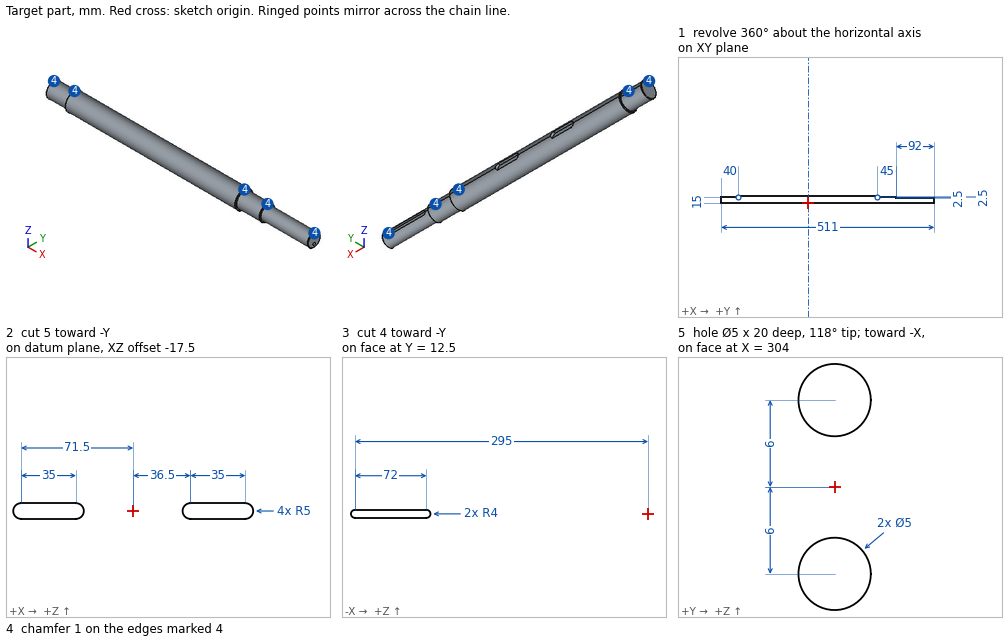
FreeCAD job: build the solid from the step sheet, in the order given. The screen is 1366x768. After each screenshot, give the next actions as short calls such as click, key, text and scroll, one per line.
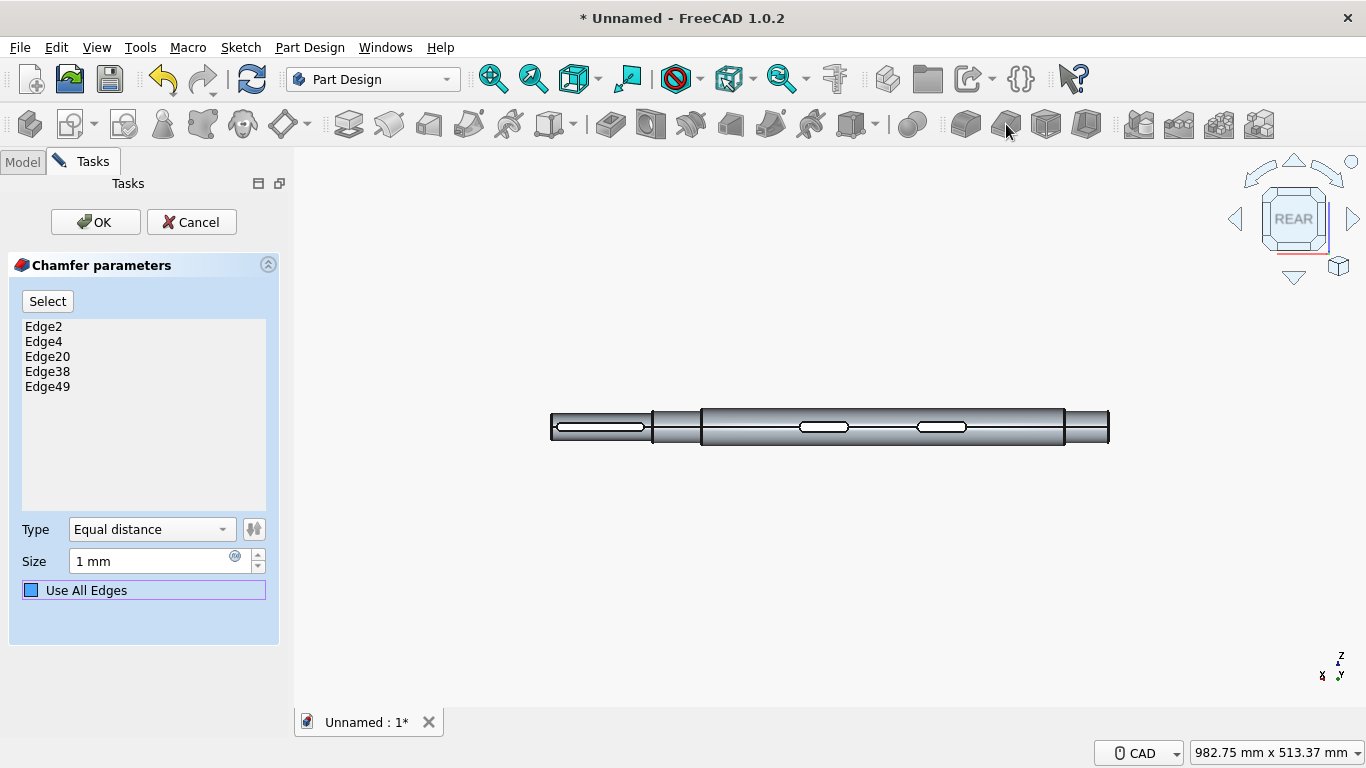
click(96, 222)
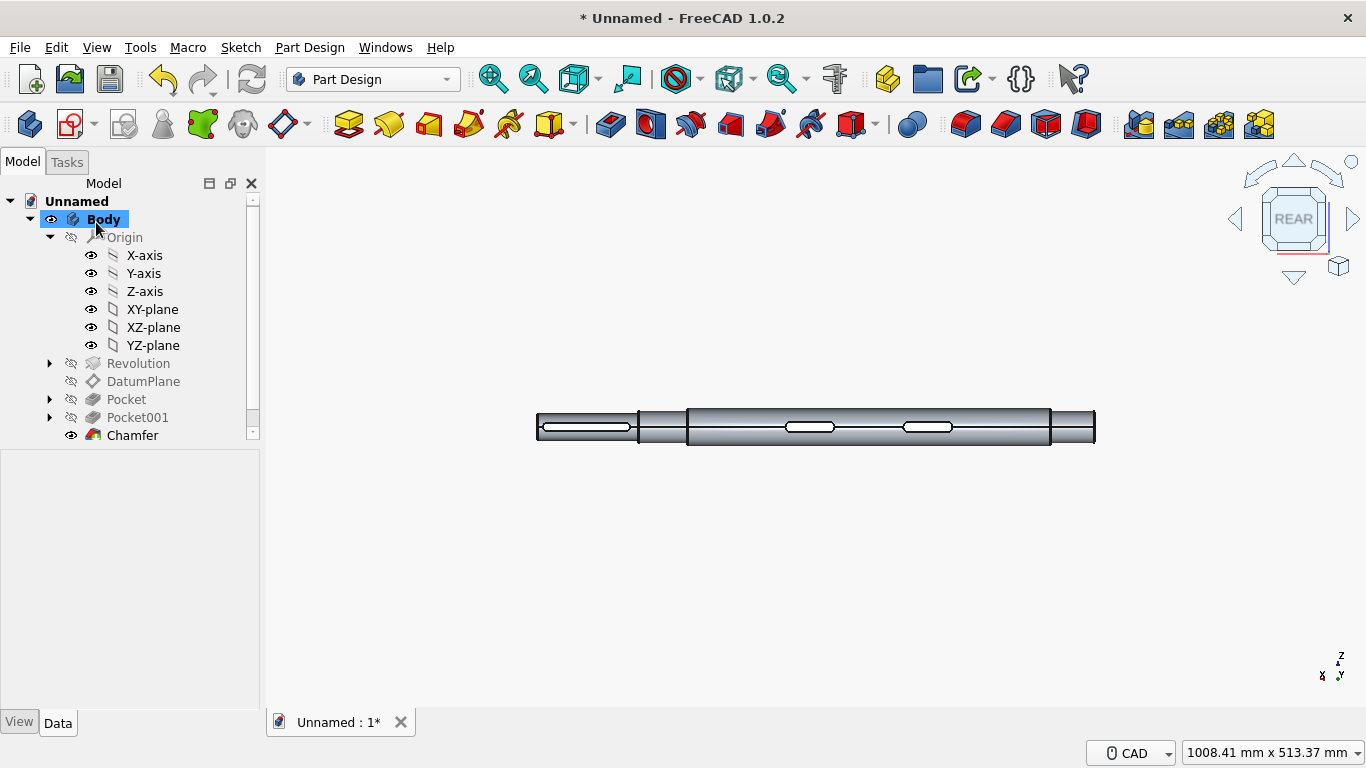
key(0)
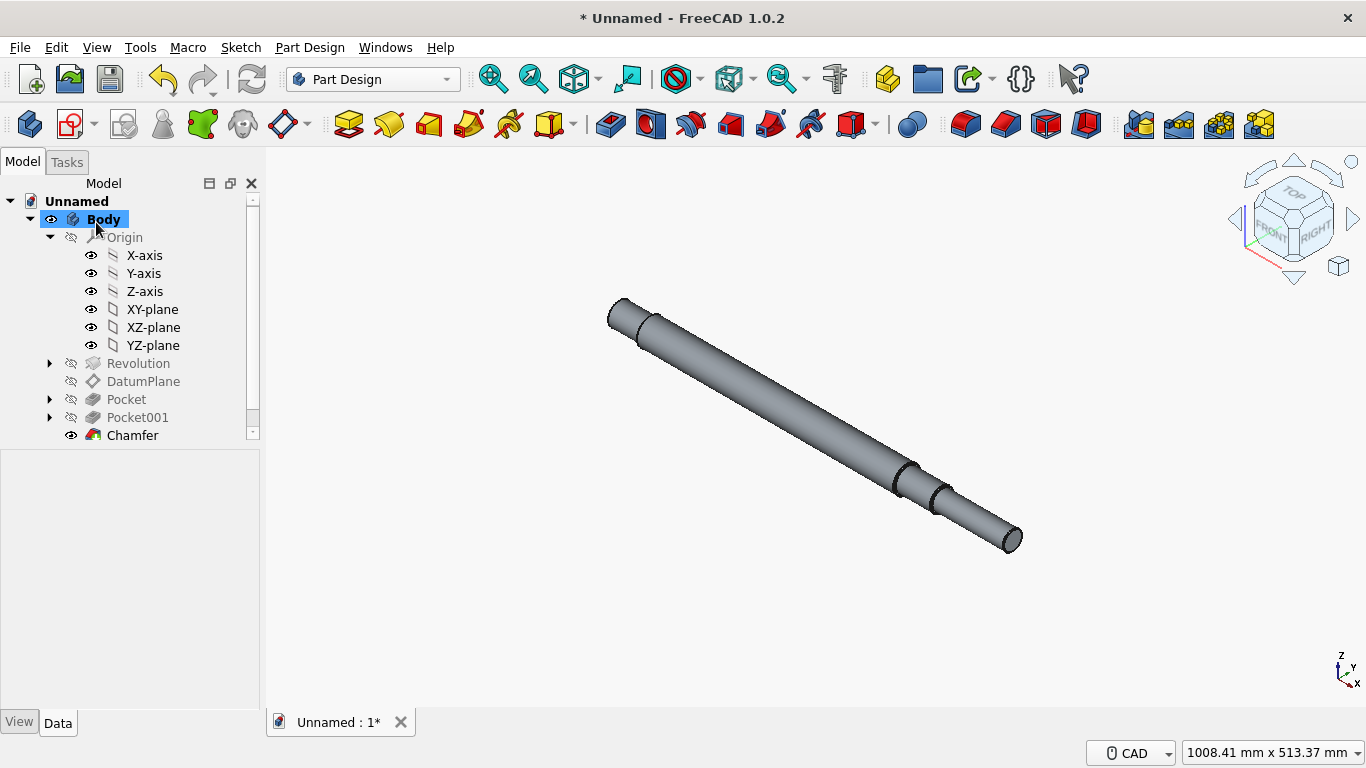
key(3)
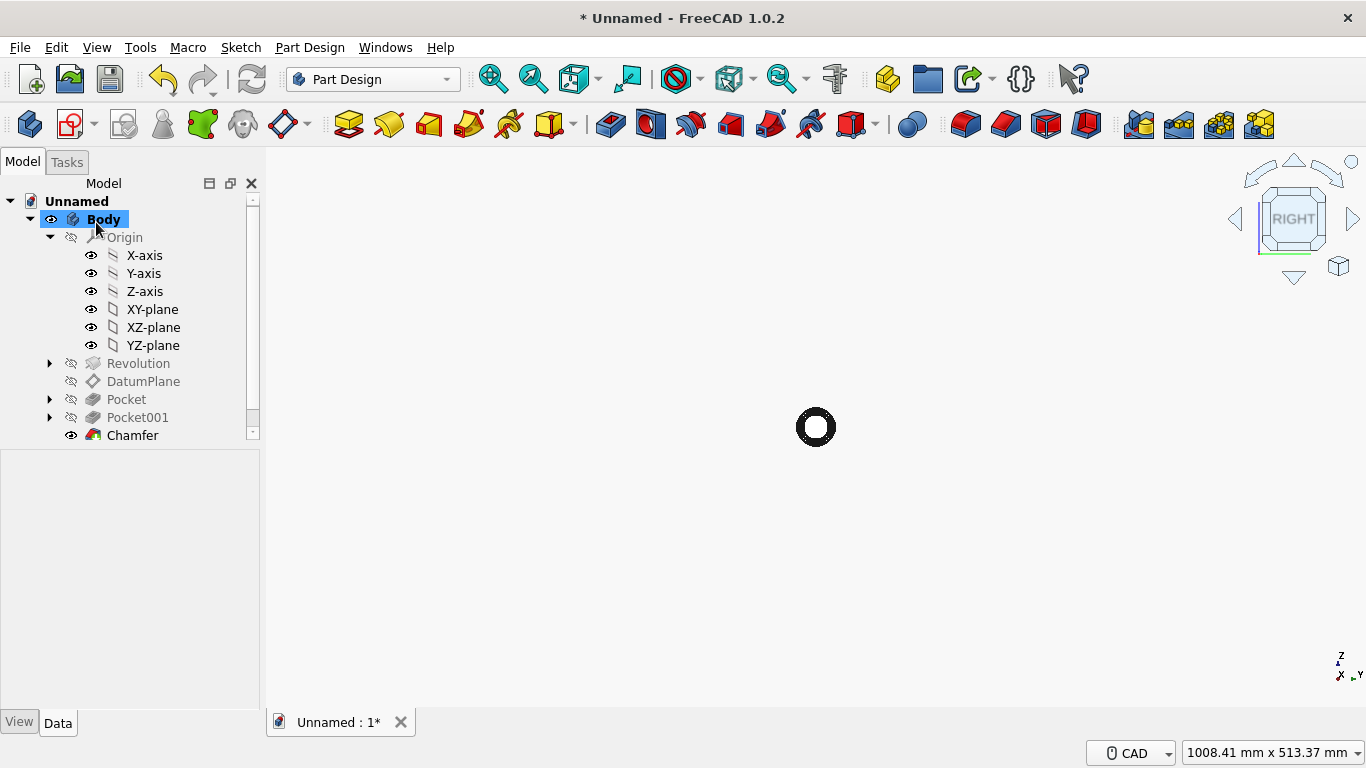
key(v)
key(f)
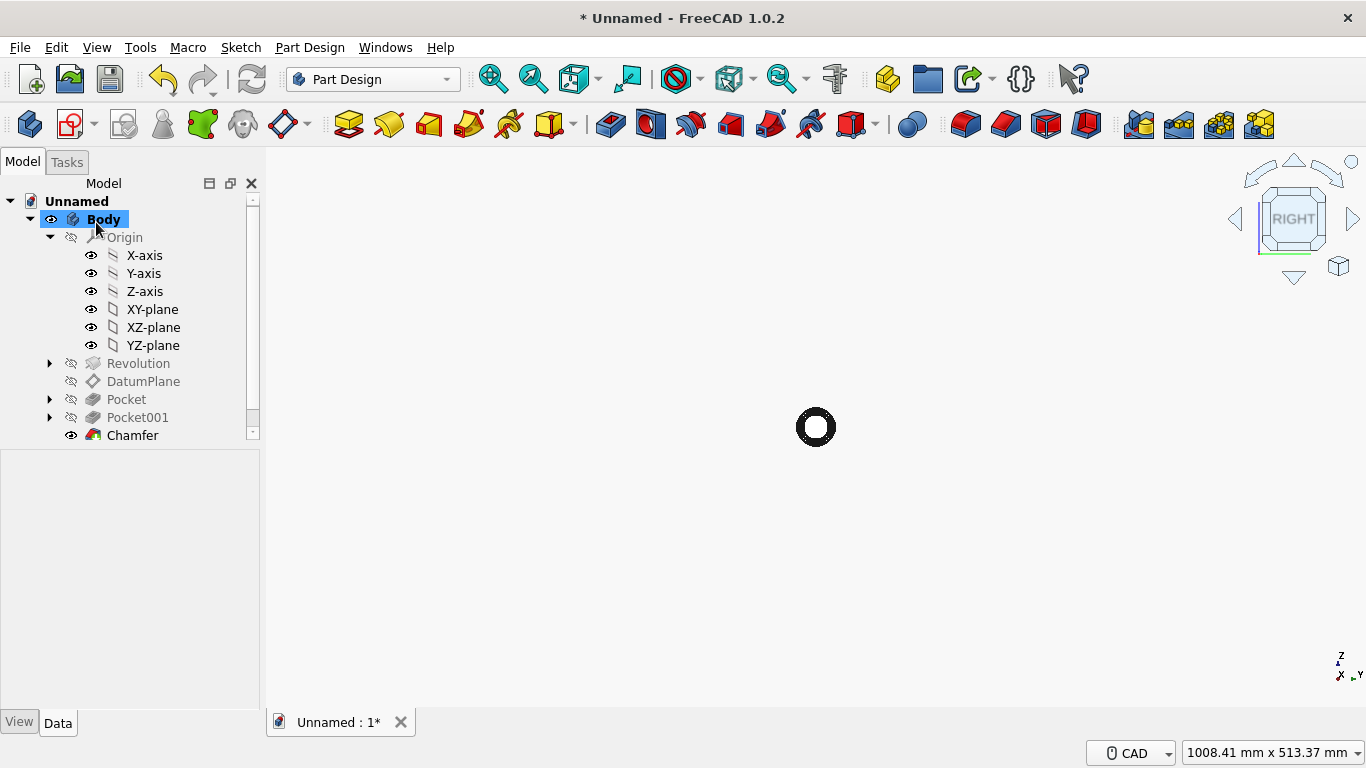
click(816, 426)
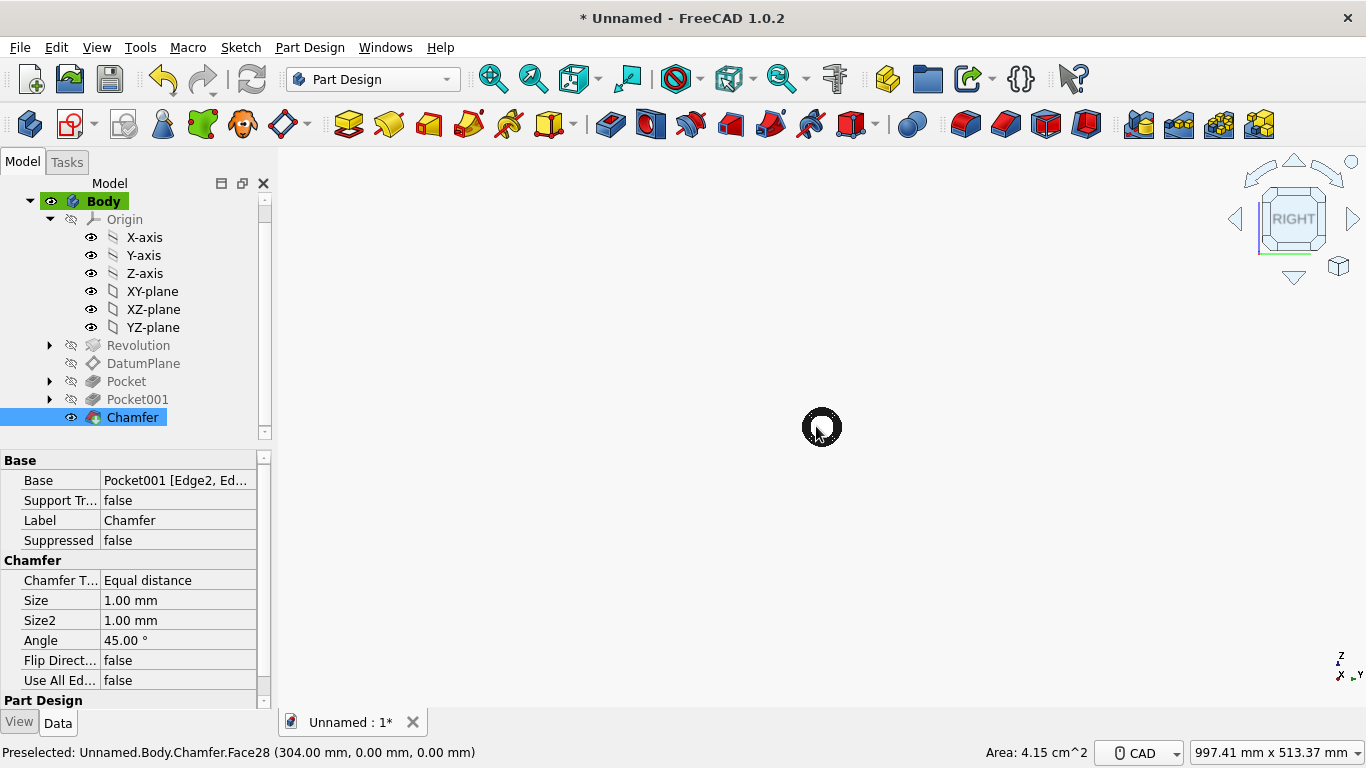
click(70, 124)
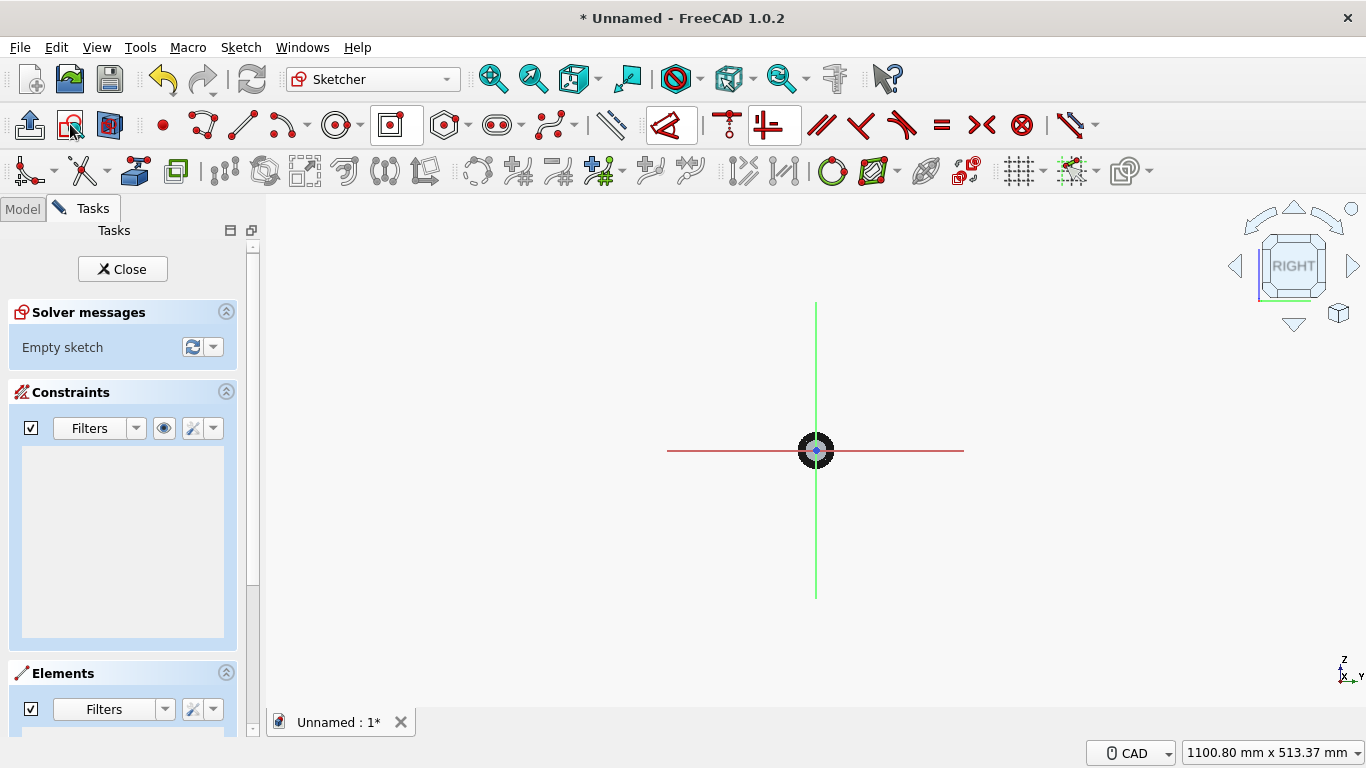
scroll(820, 451, up, 15)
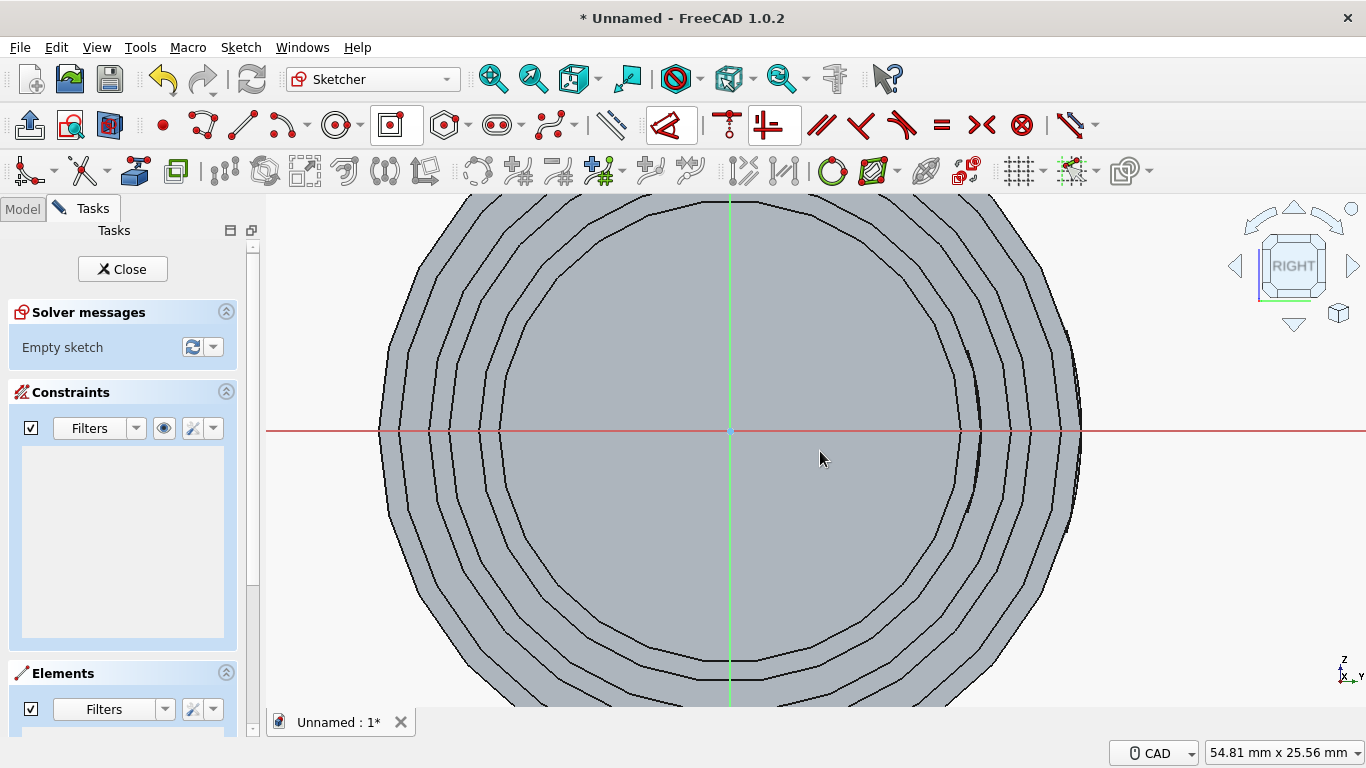
key(g)
key(c)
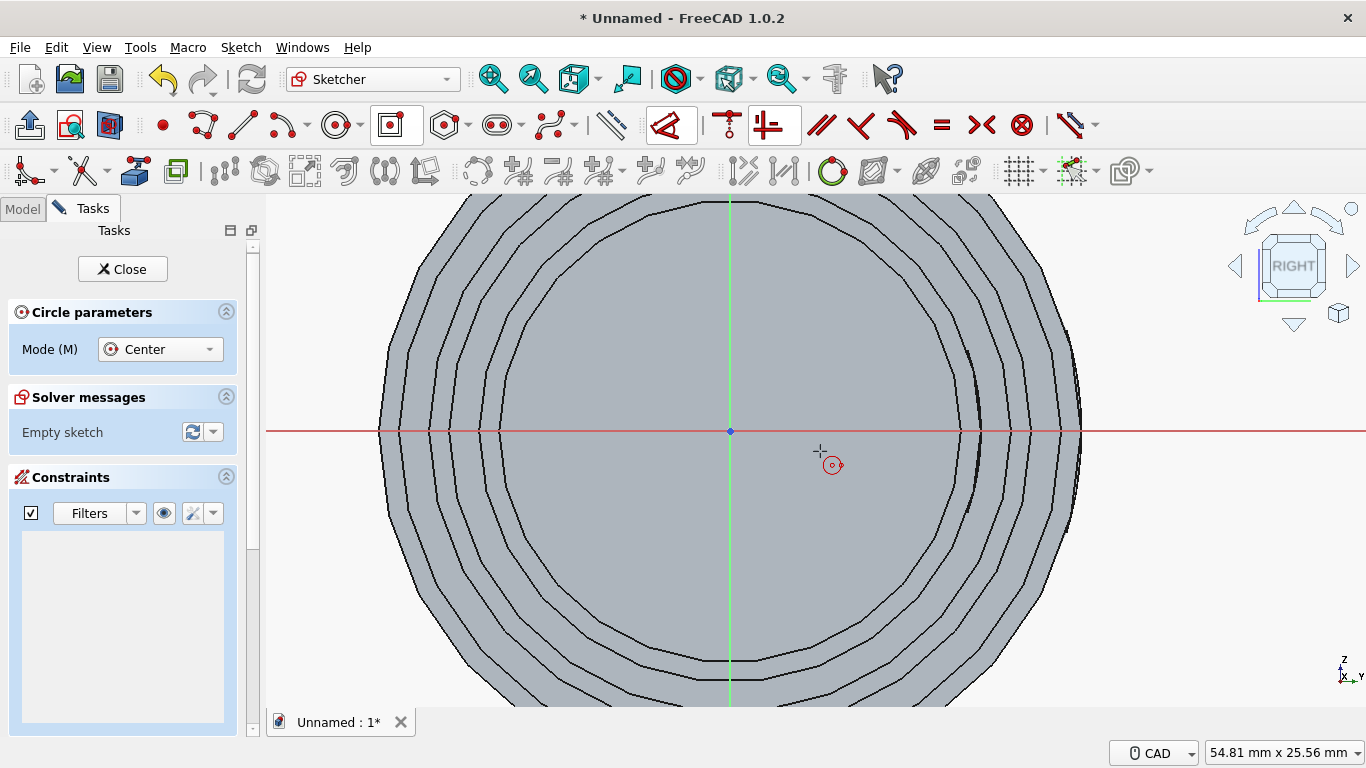
click(730, 552)
click(766, 516)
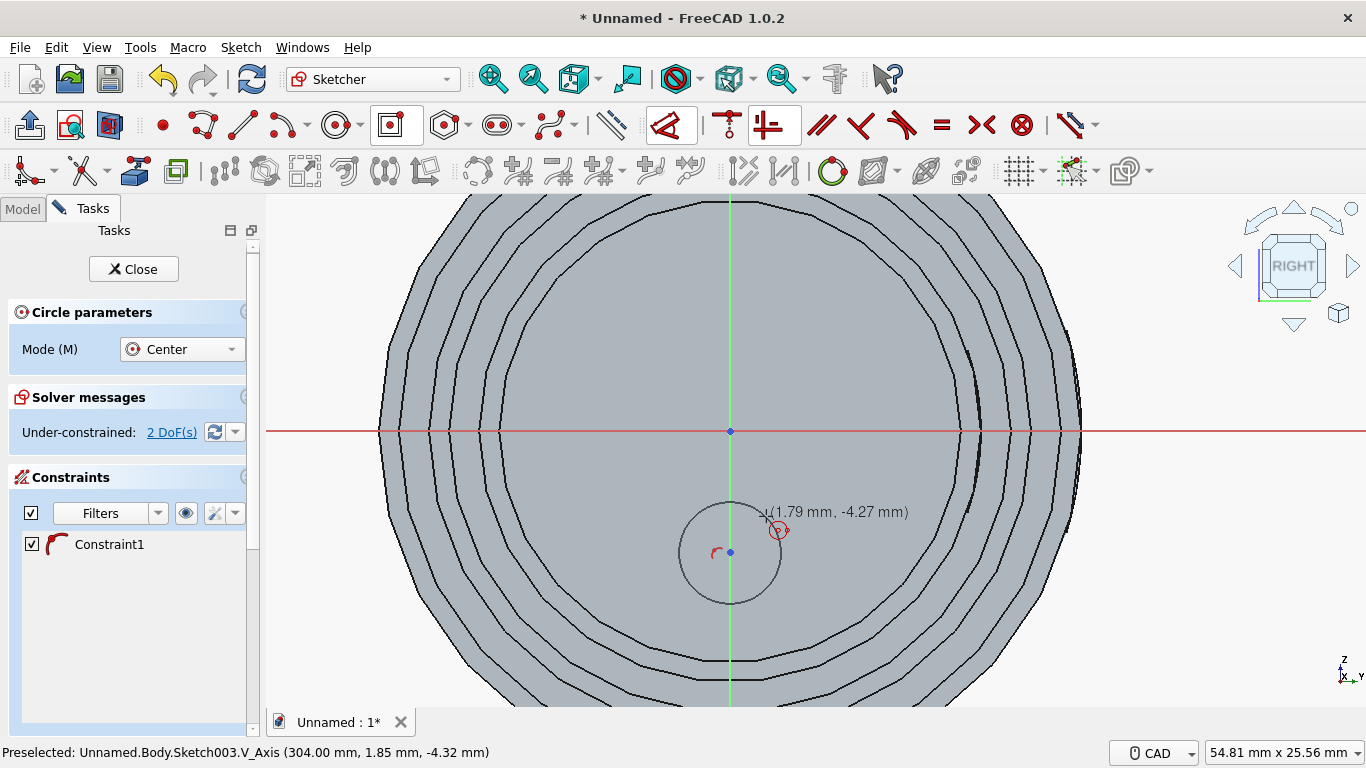
click(730, 311)
click(766, 275)
key(Escape)